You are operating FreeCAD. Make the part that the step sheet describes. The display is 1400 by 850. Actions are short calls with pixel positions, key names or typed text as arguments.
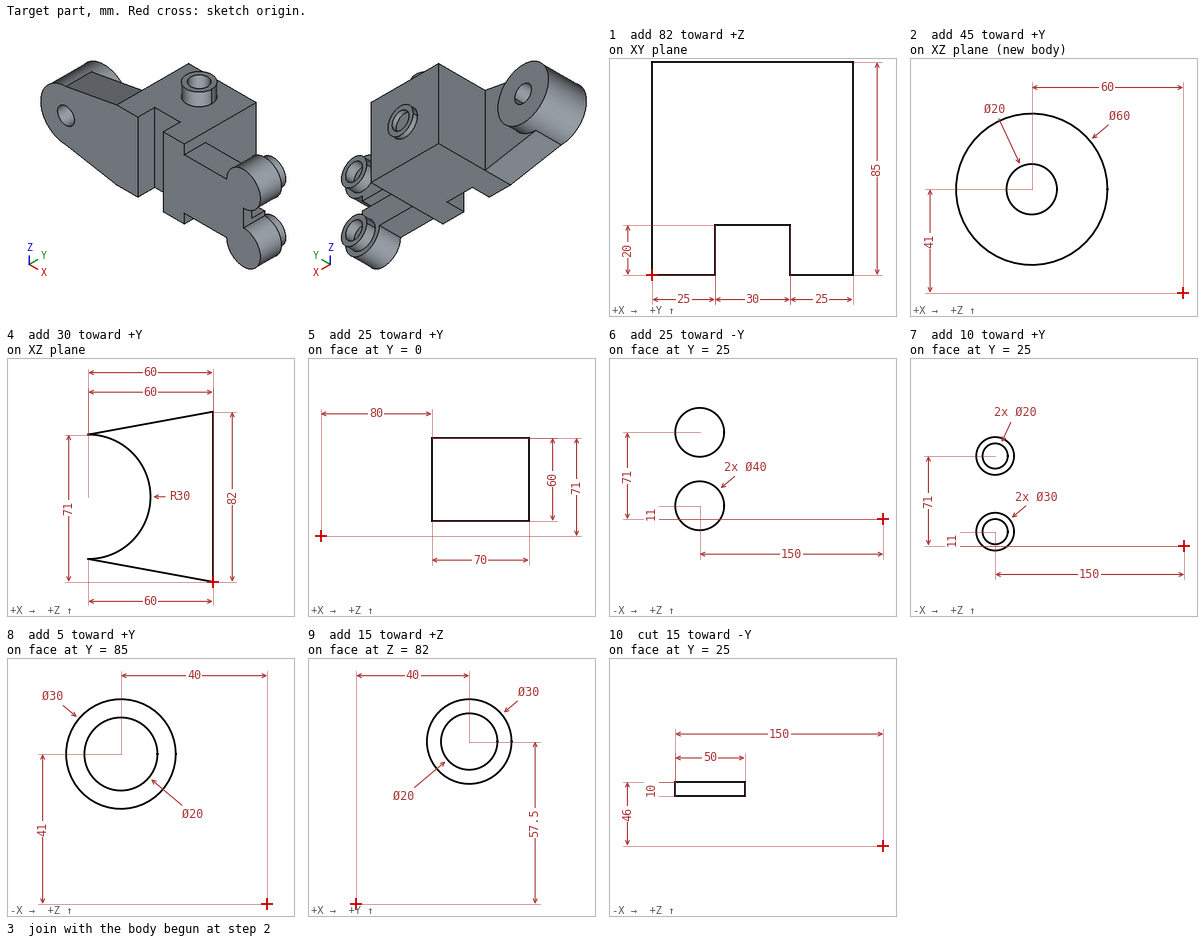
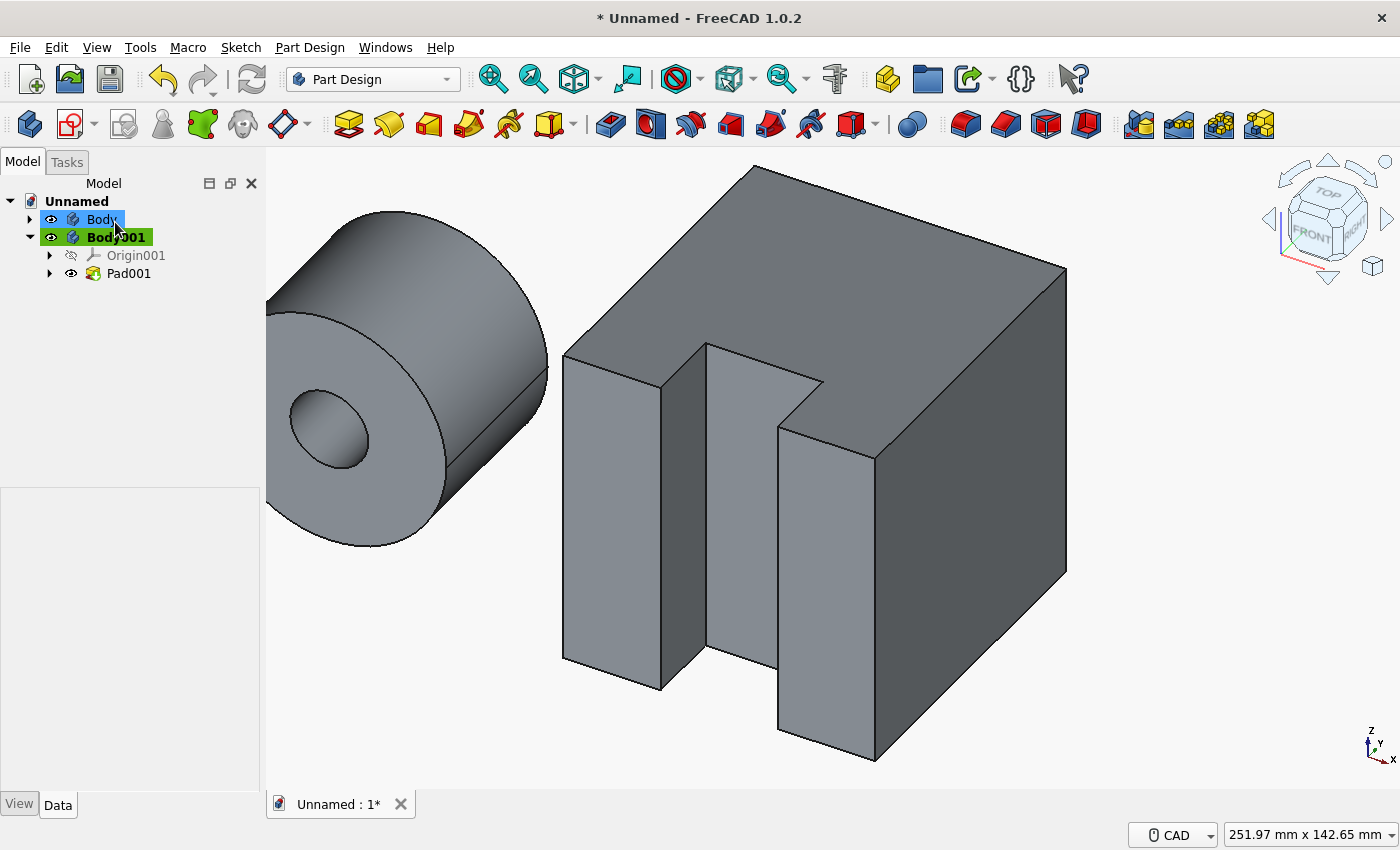
click(494, 80)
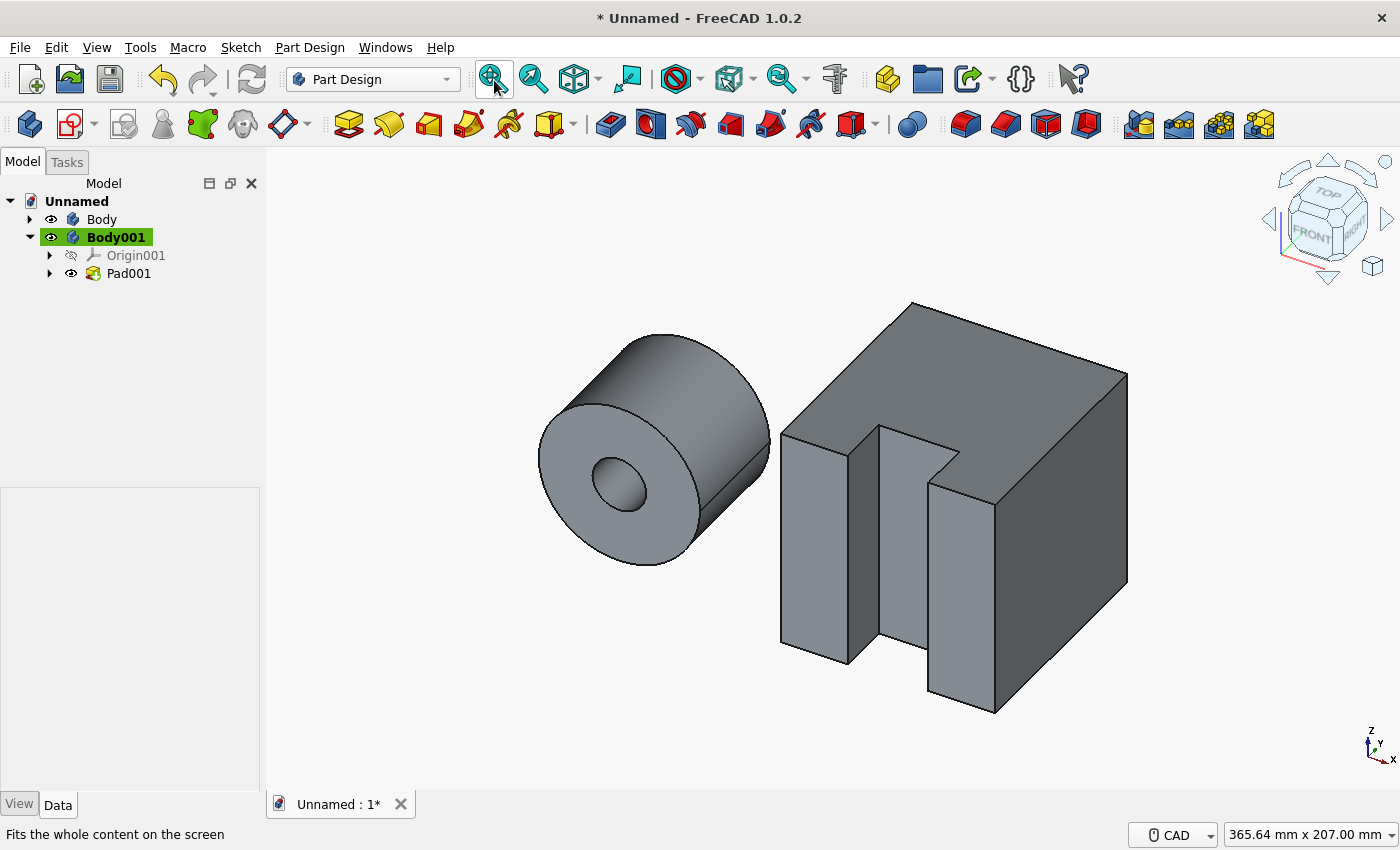
double_click(96, 219)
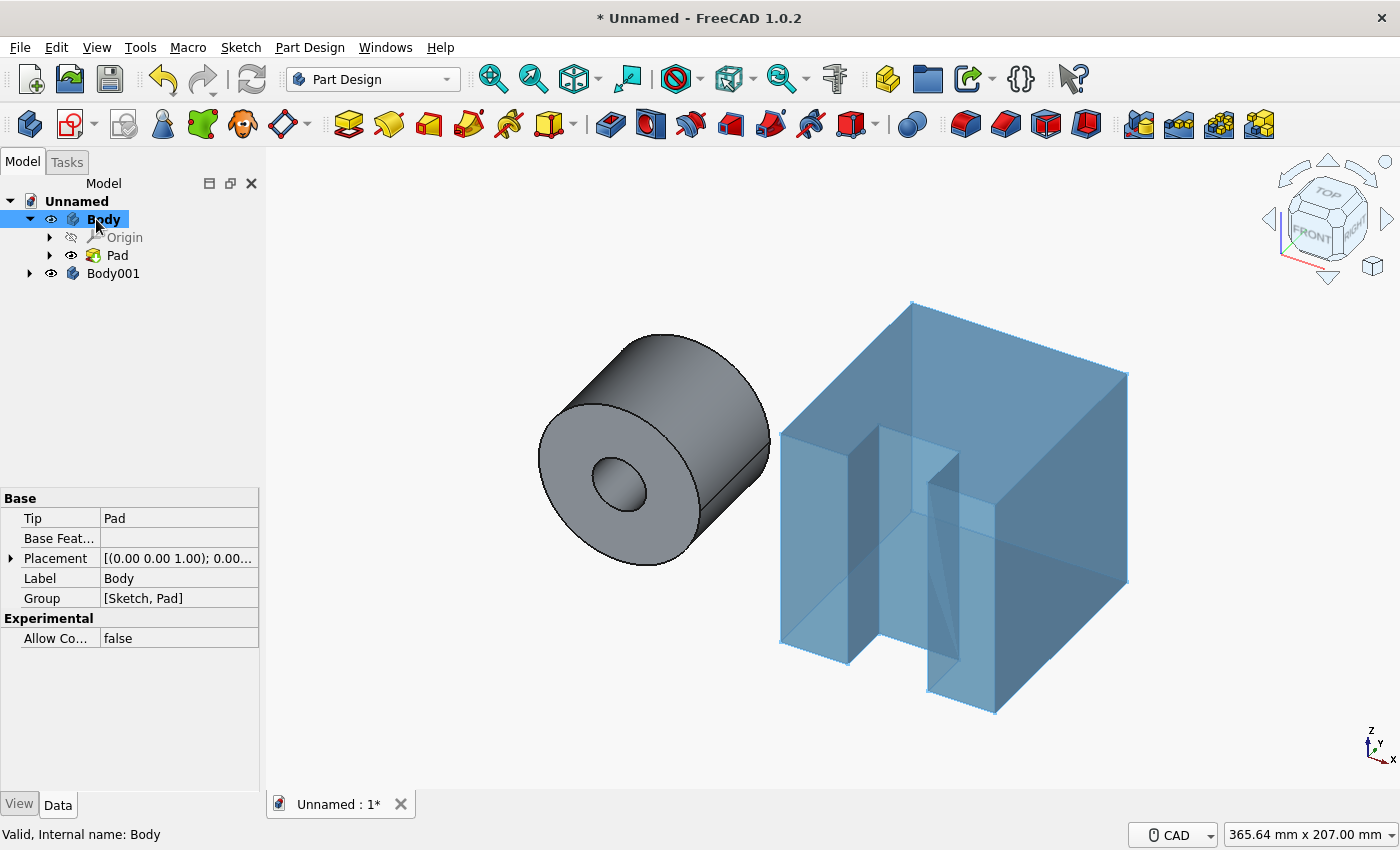
click(96, 219)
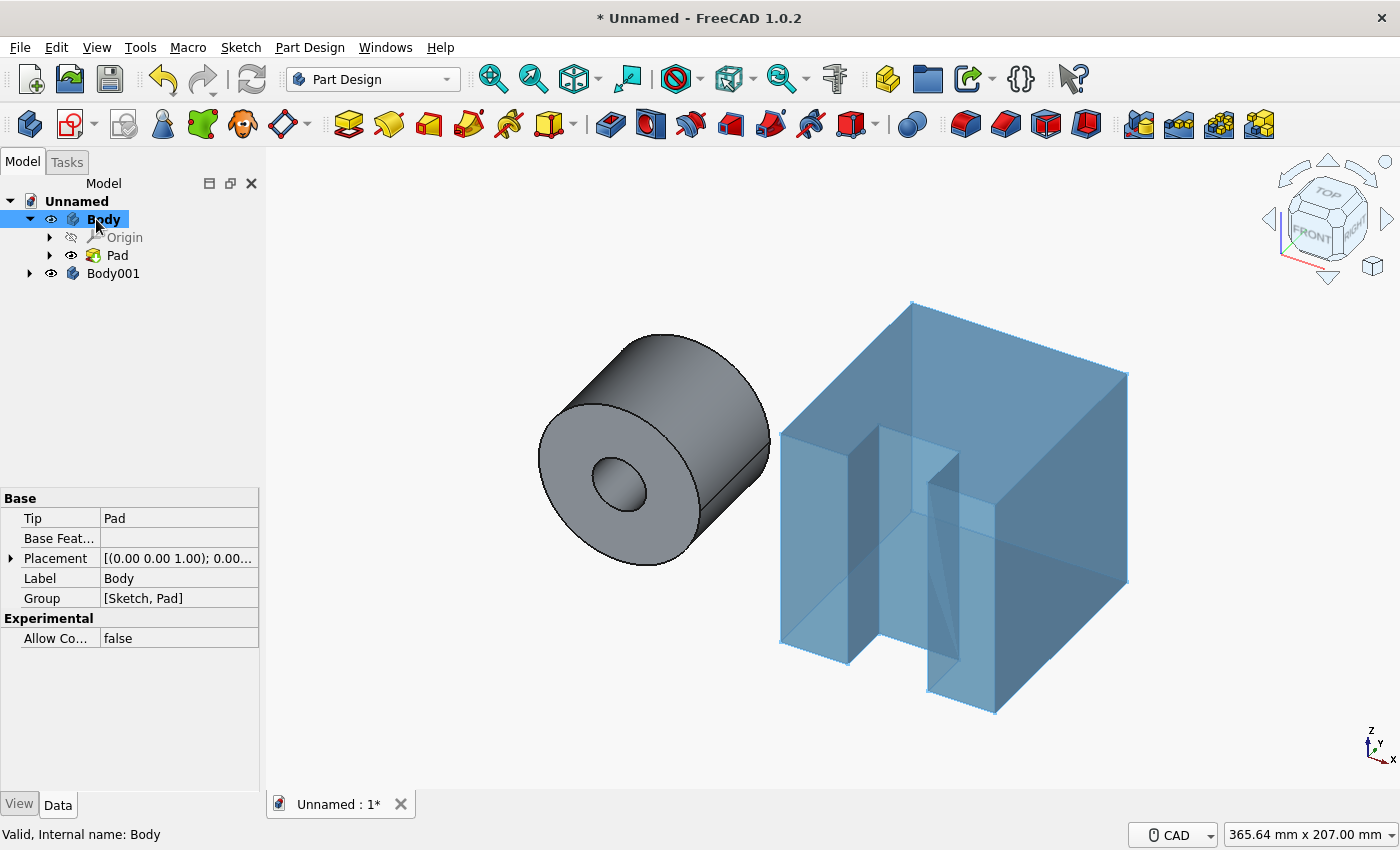
click(146, 638)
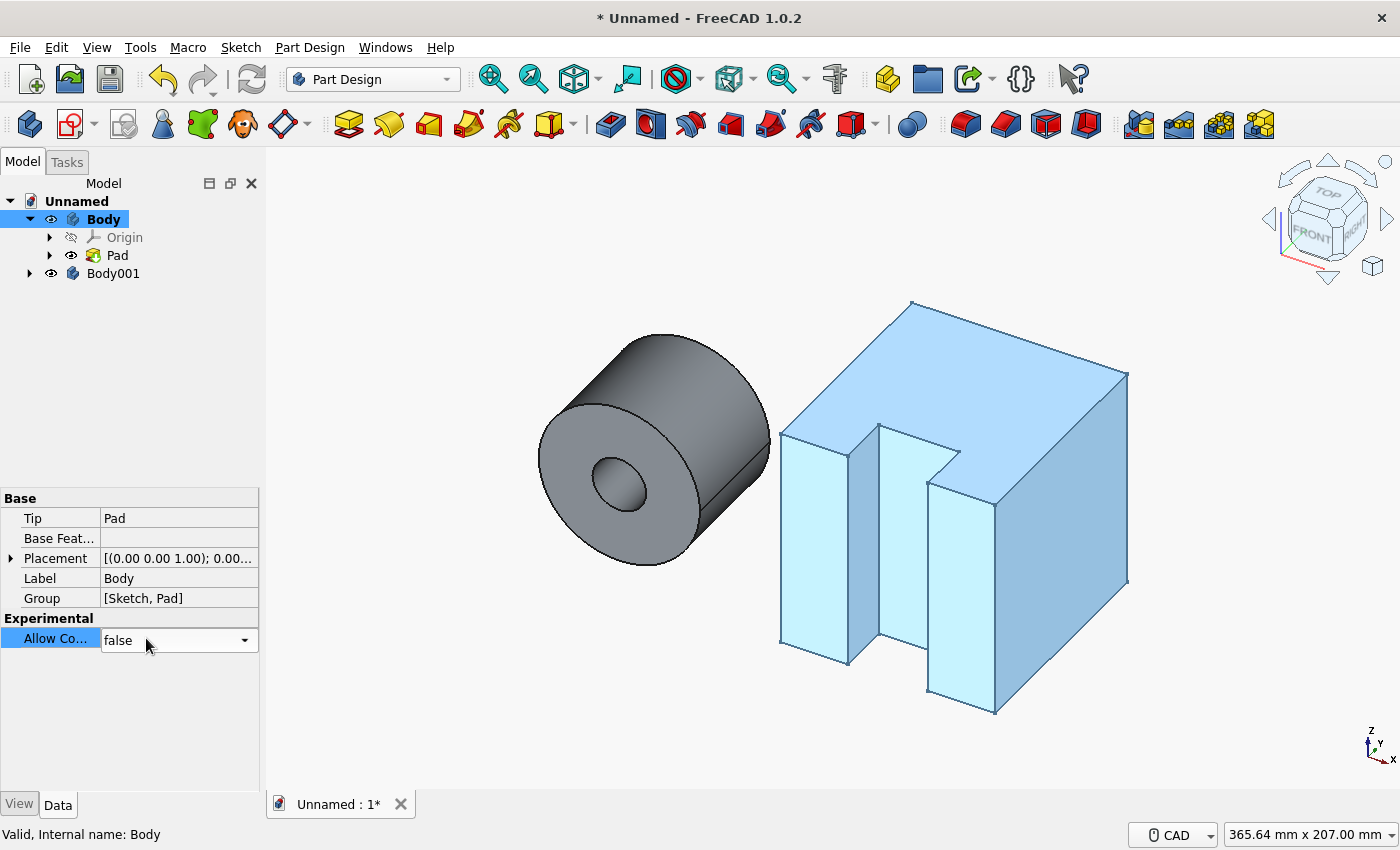
click(146, 638)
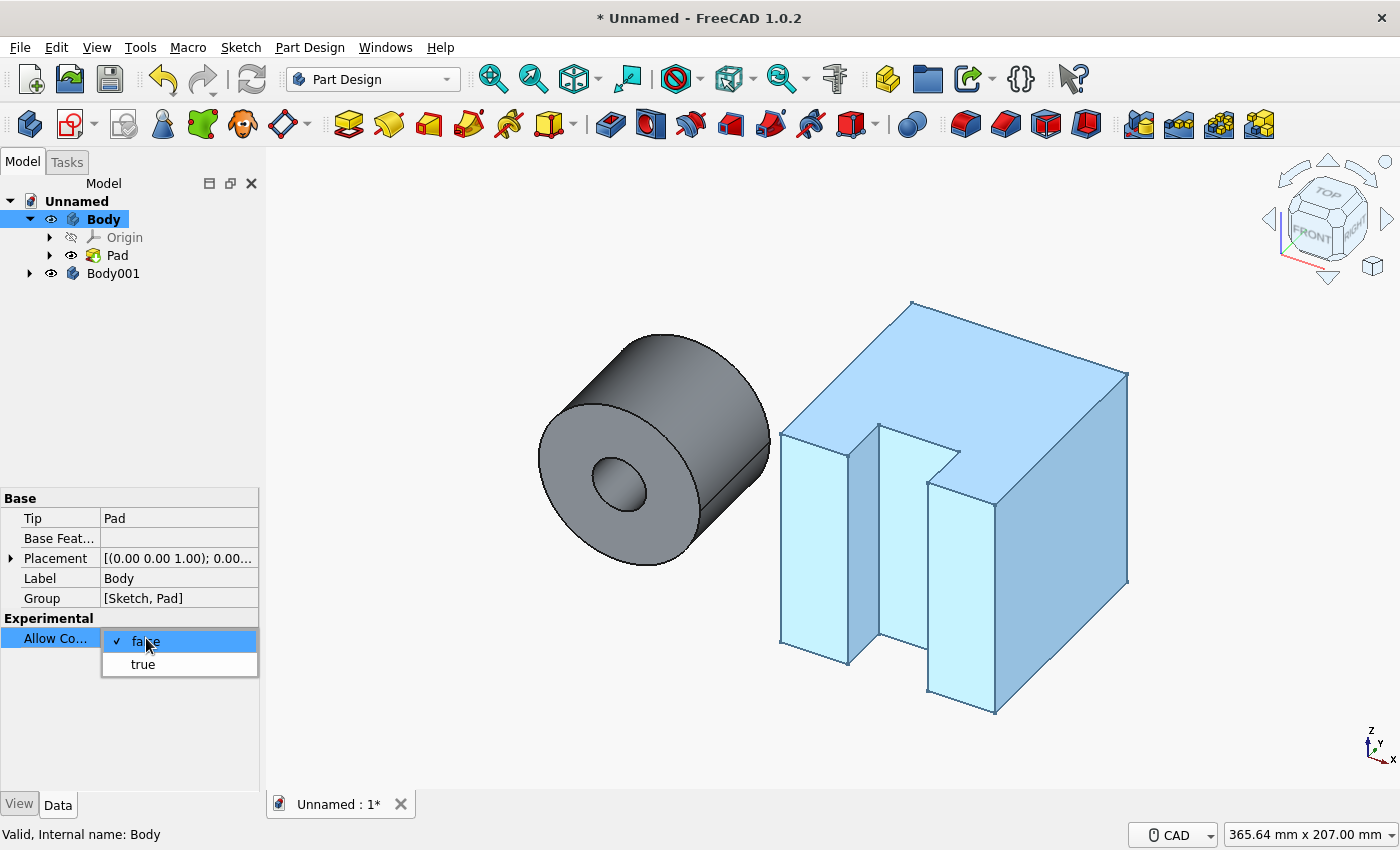
click(179, 664)
key(Return)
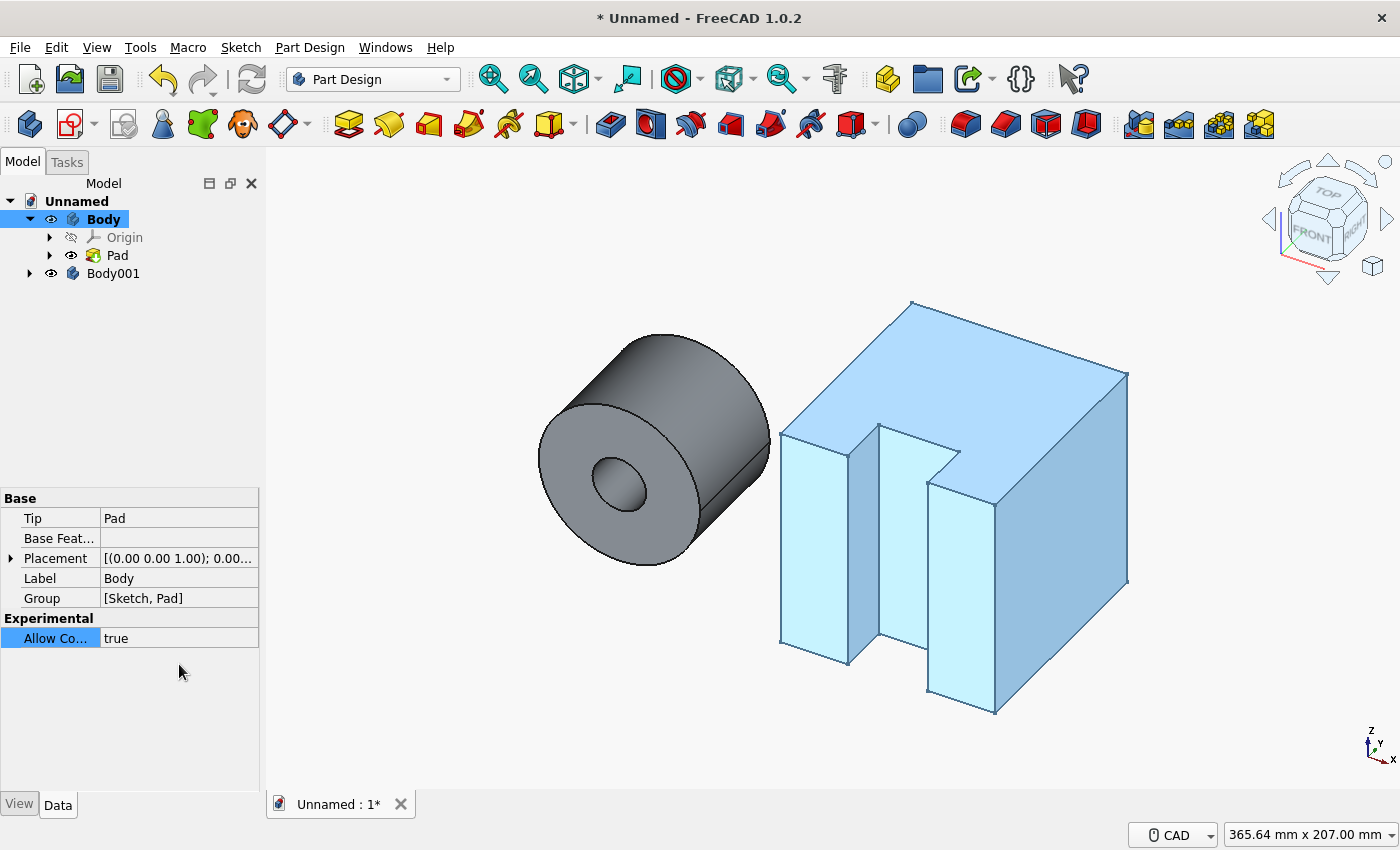
click(96, 273)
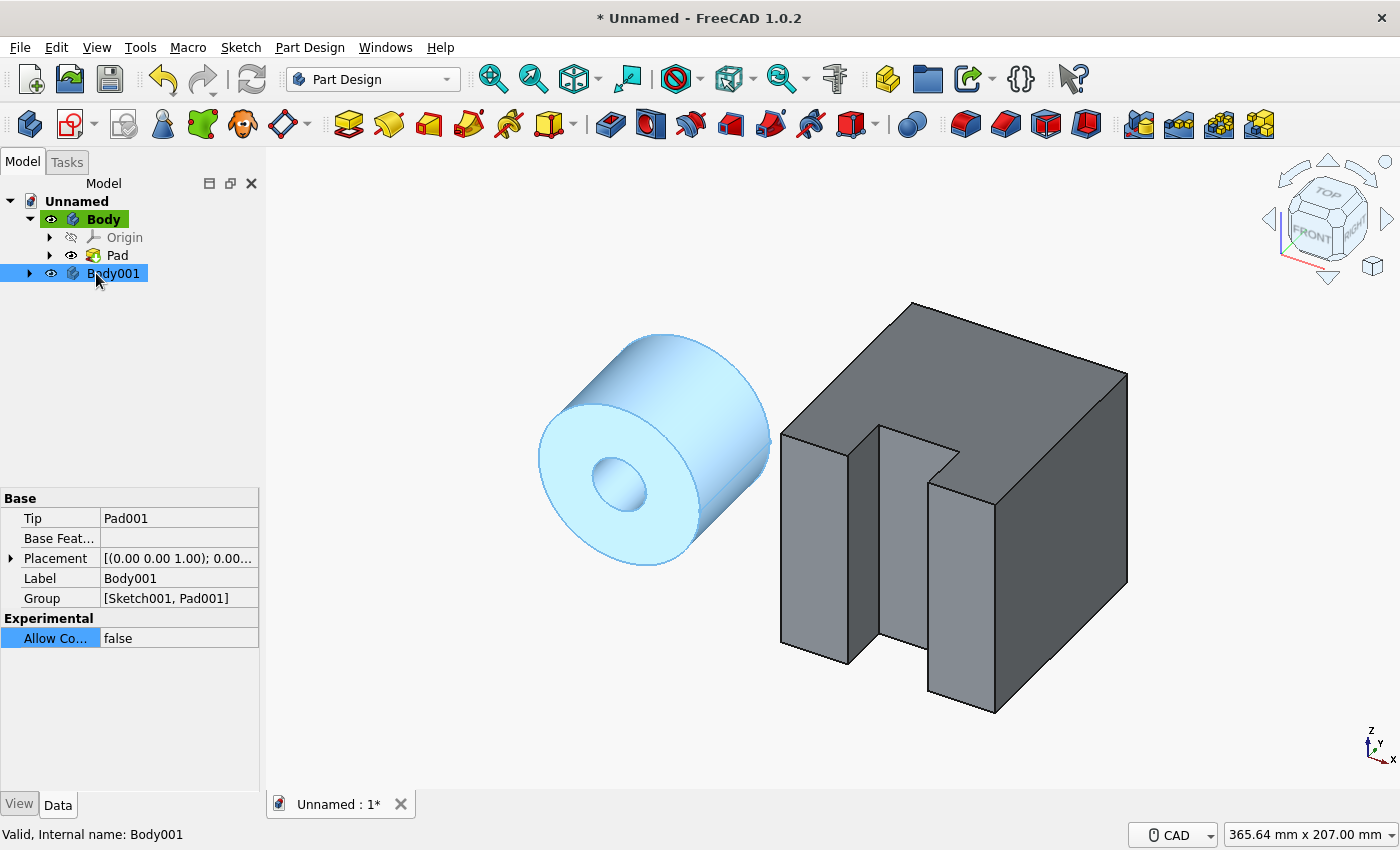
click(914, 124)